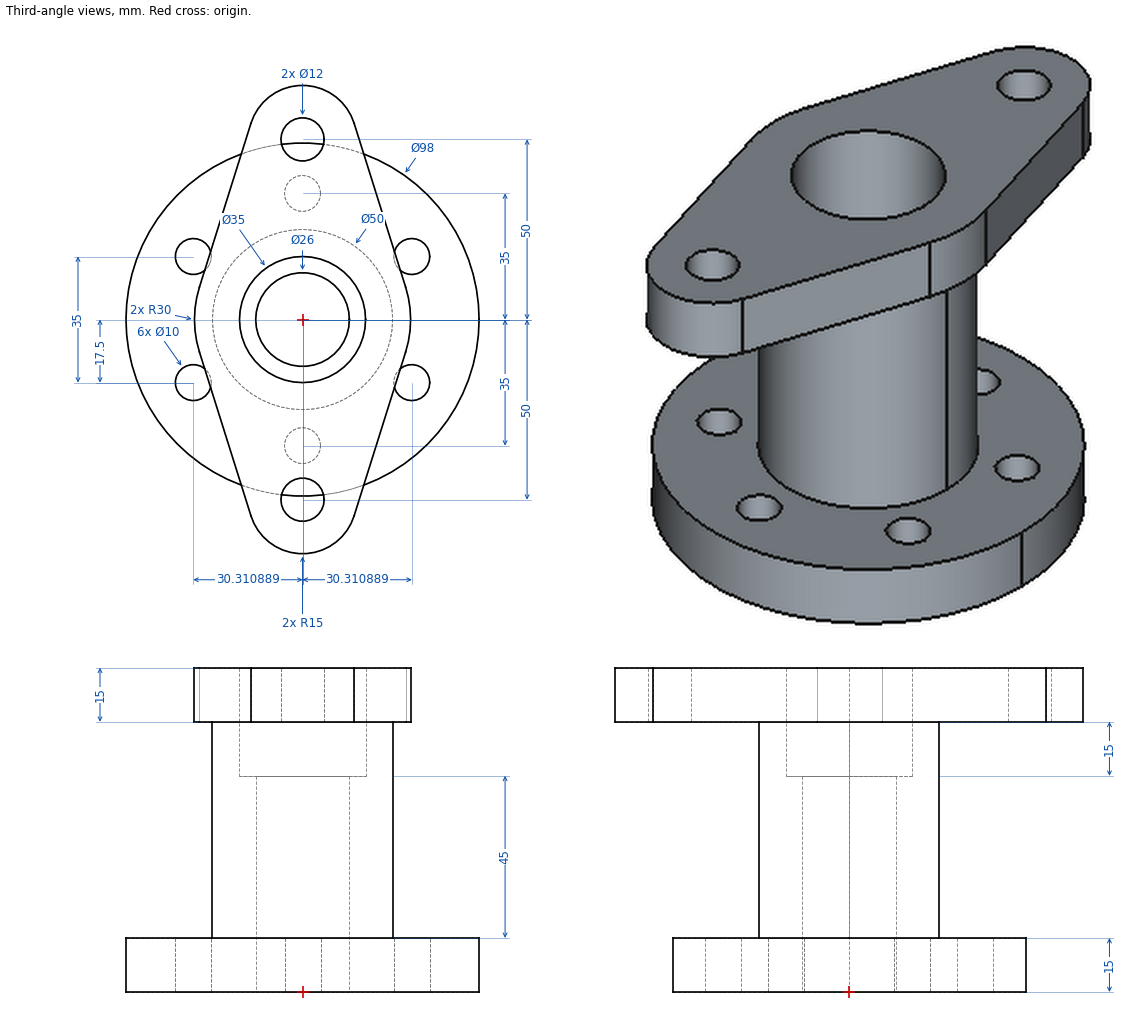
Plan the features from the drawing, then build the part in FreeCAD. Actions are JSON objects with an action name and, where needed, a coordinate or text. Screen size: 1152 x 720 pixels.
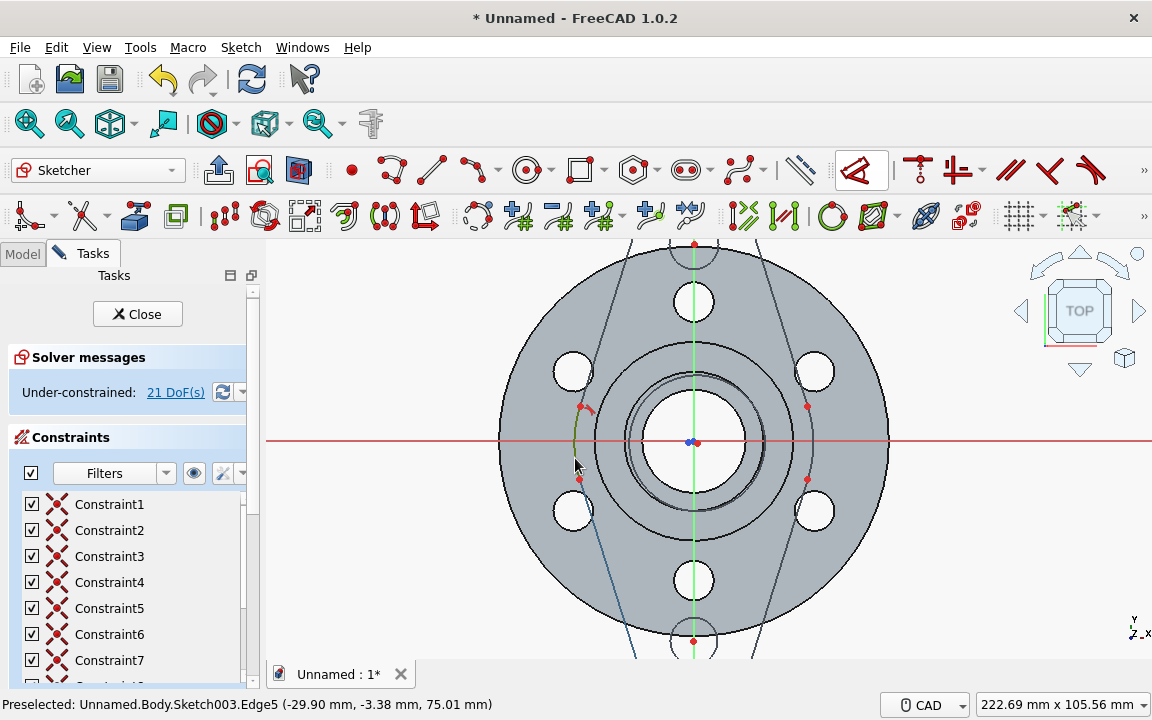
{"action": "left_click", "coordinate": [1092, 170]}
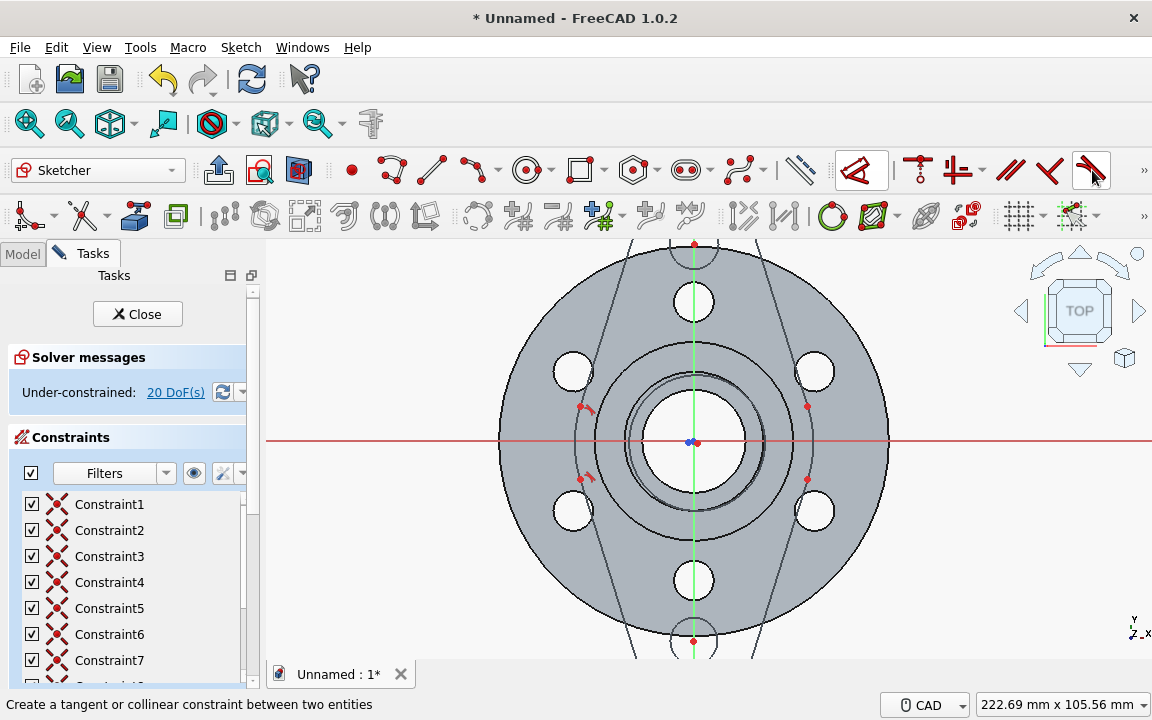
{"action": "left_click", "coordinate": [597, 534]}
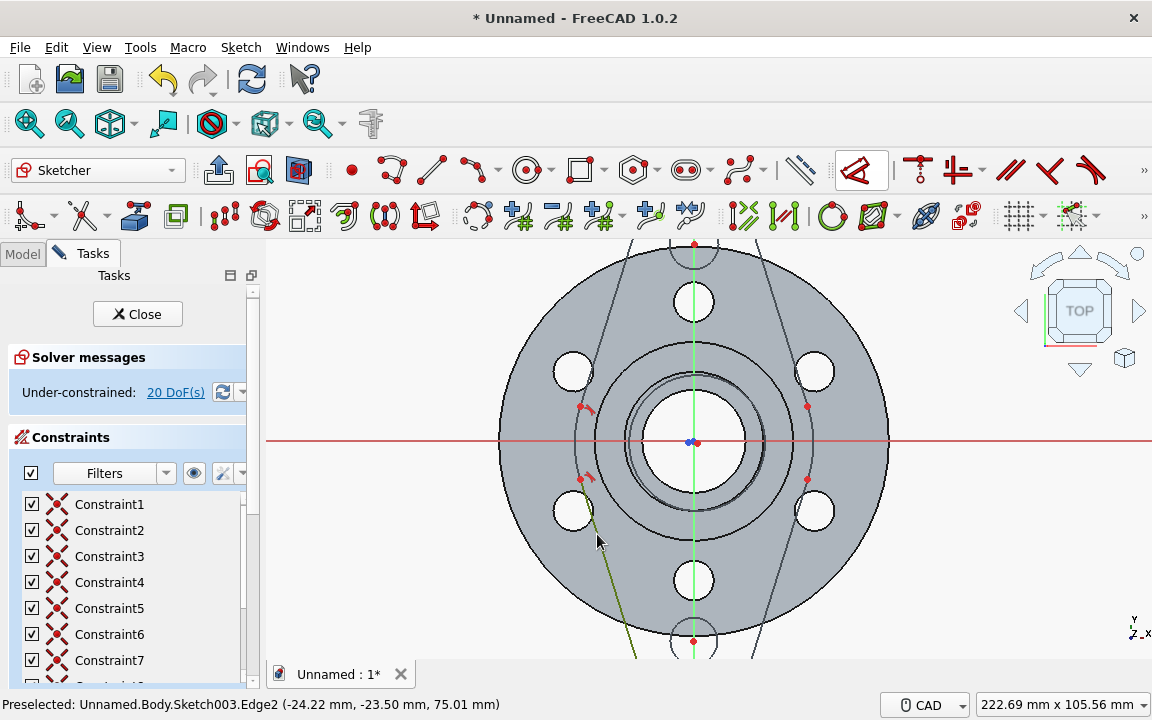
{"action": "scroll", "coordinate": [576, 458], "scroll_direction": "down", "scroll_amount": 3}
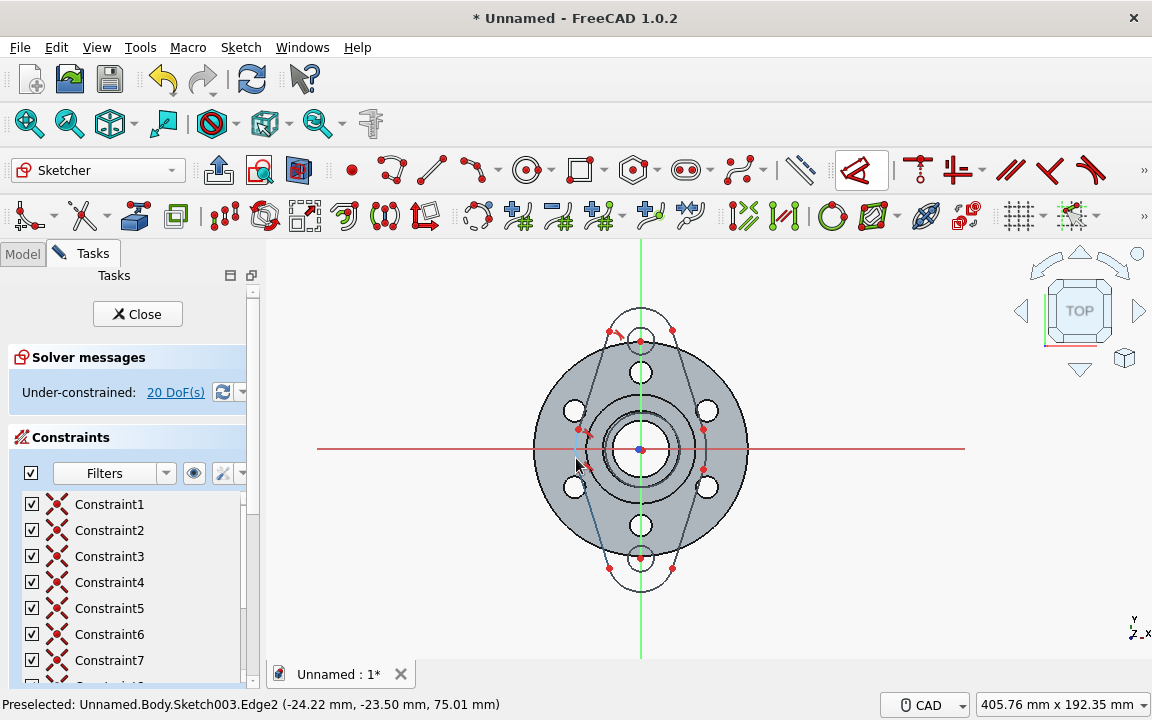
{"action": "left_click", "coordinate": [625, 588]}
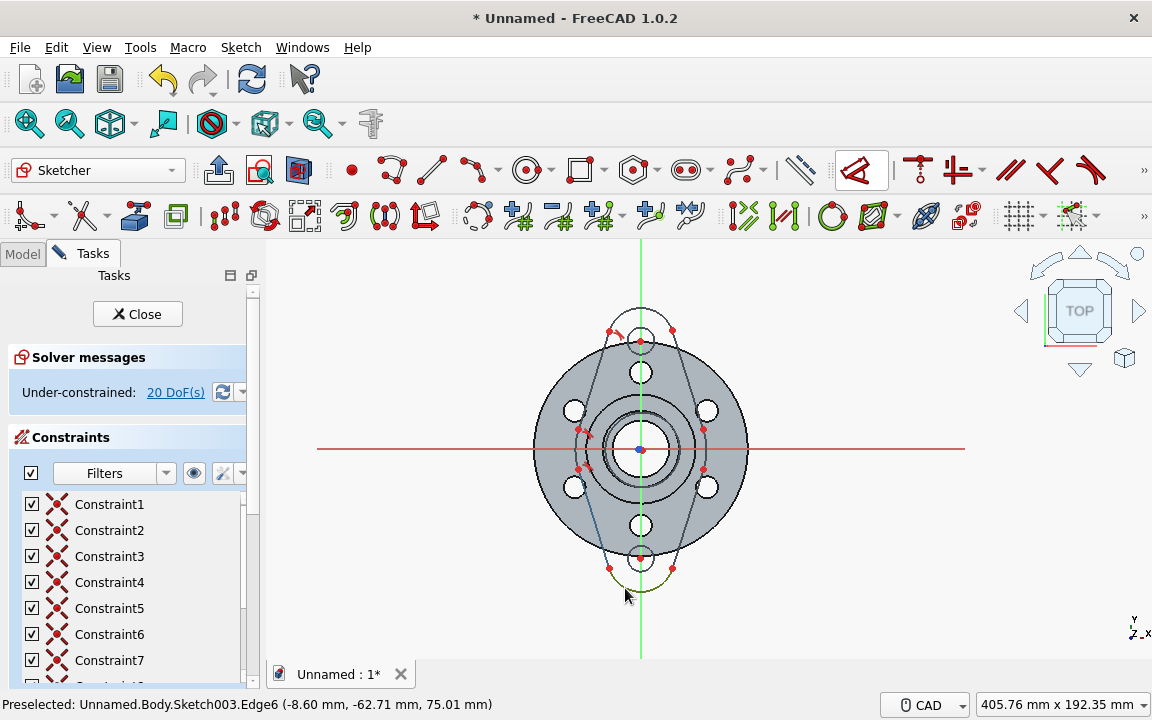
{"action": "key", "text": "t"}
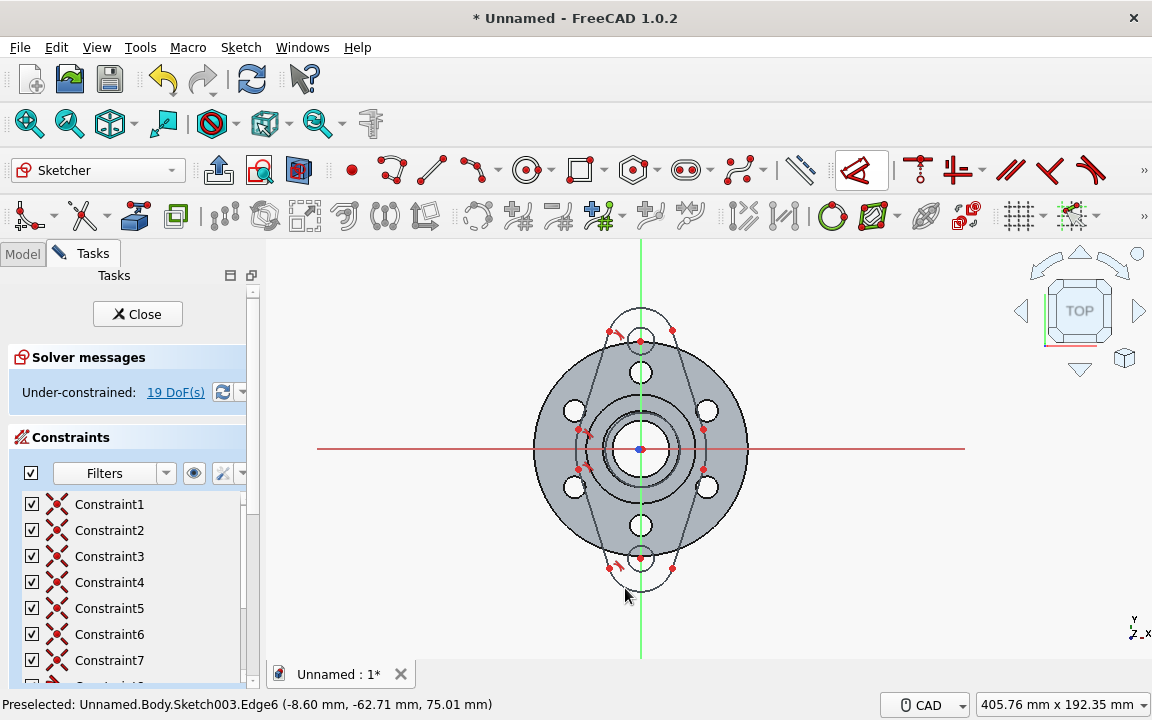
{"action": "left_click", "coordinate": [682, 539]}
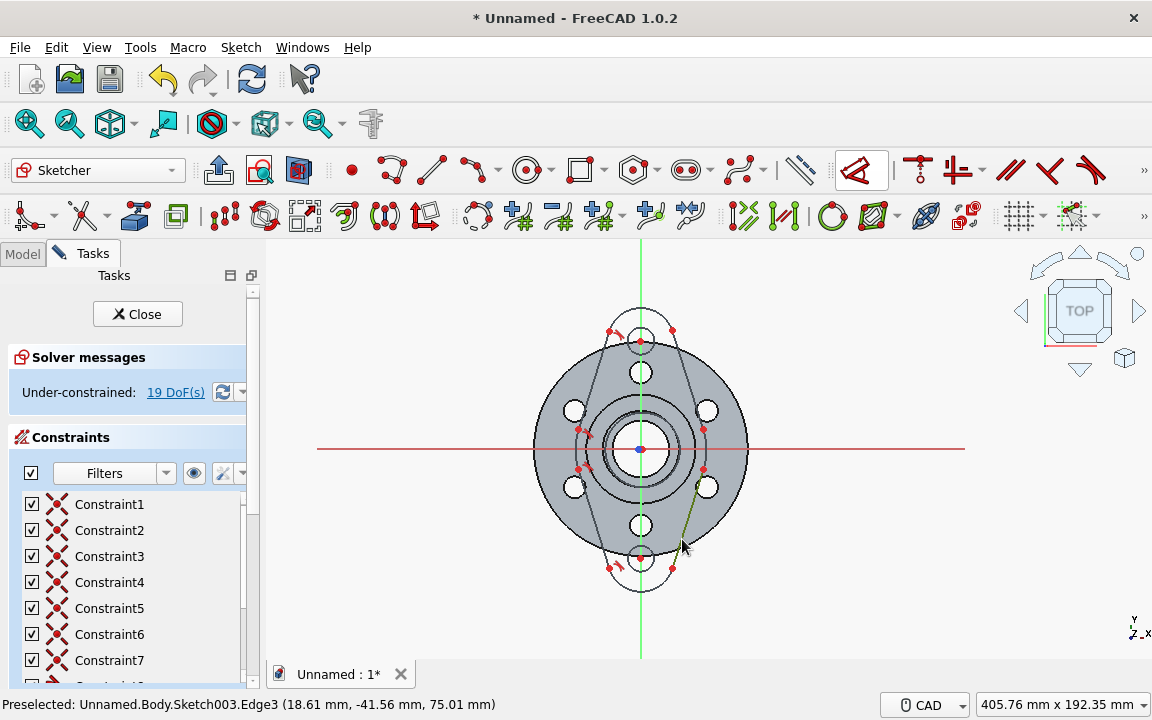
{"action": "left_click", "coordinate": [625, 588]}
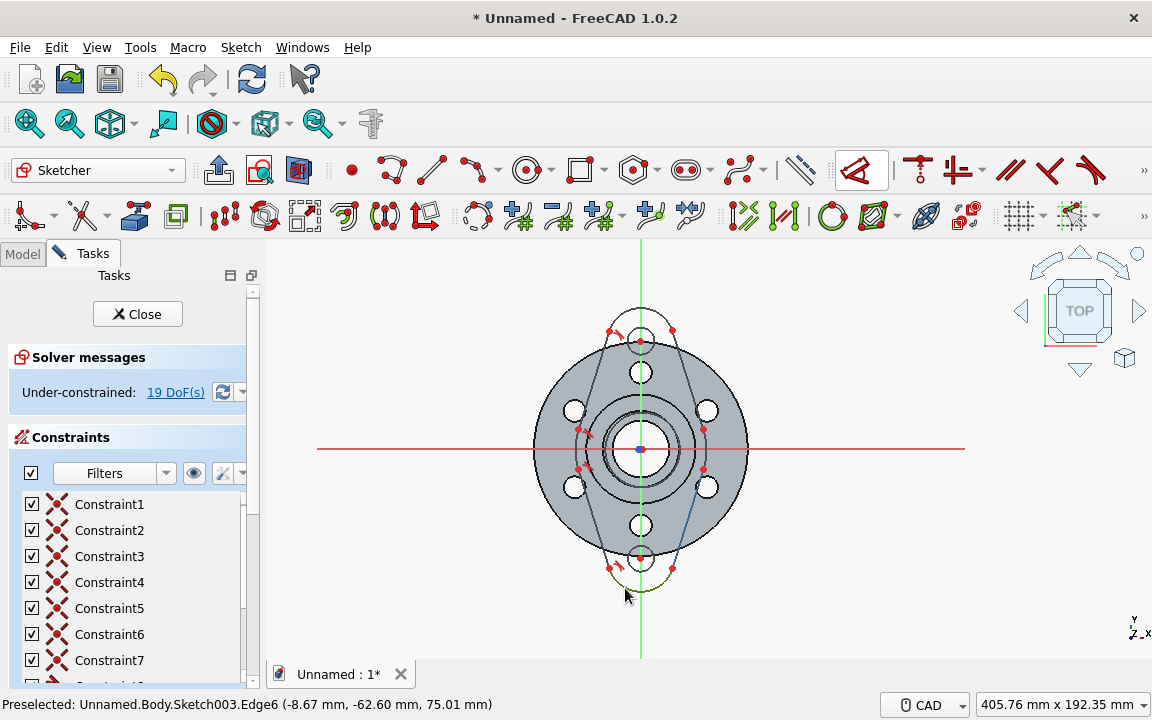
{"action": "key", "text": "t"}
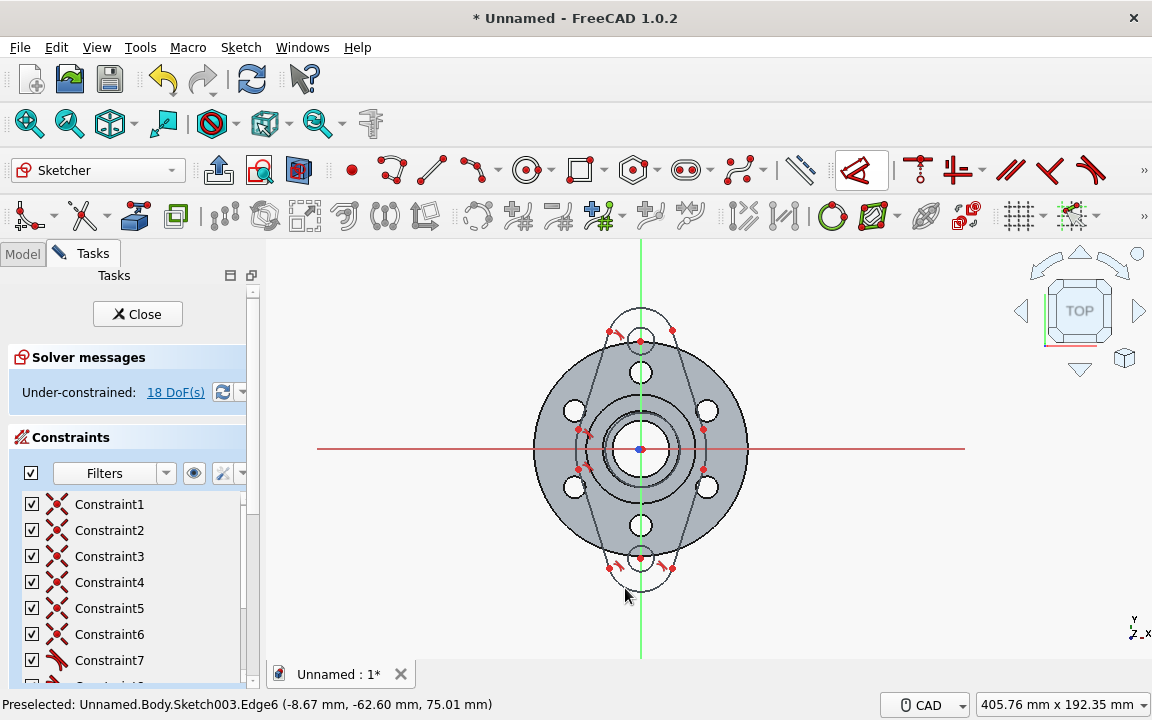
{"action": "left_click", "coordinate": [682, 539]}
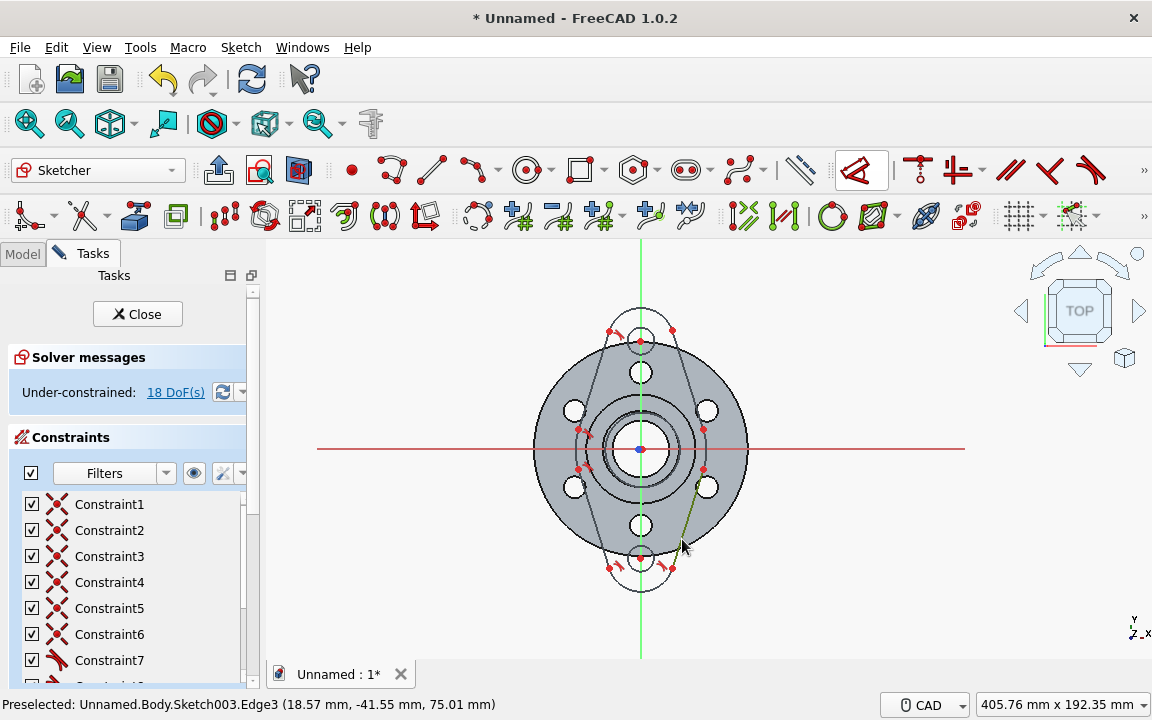
{"action": "scroll", "coordinate": [706, 458], "scroll_direction": "up", "scroll_amount": 3}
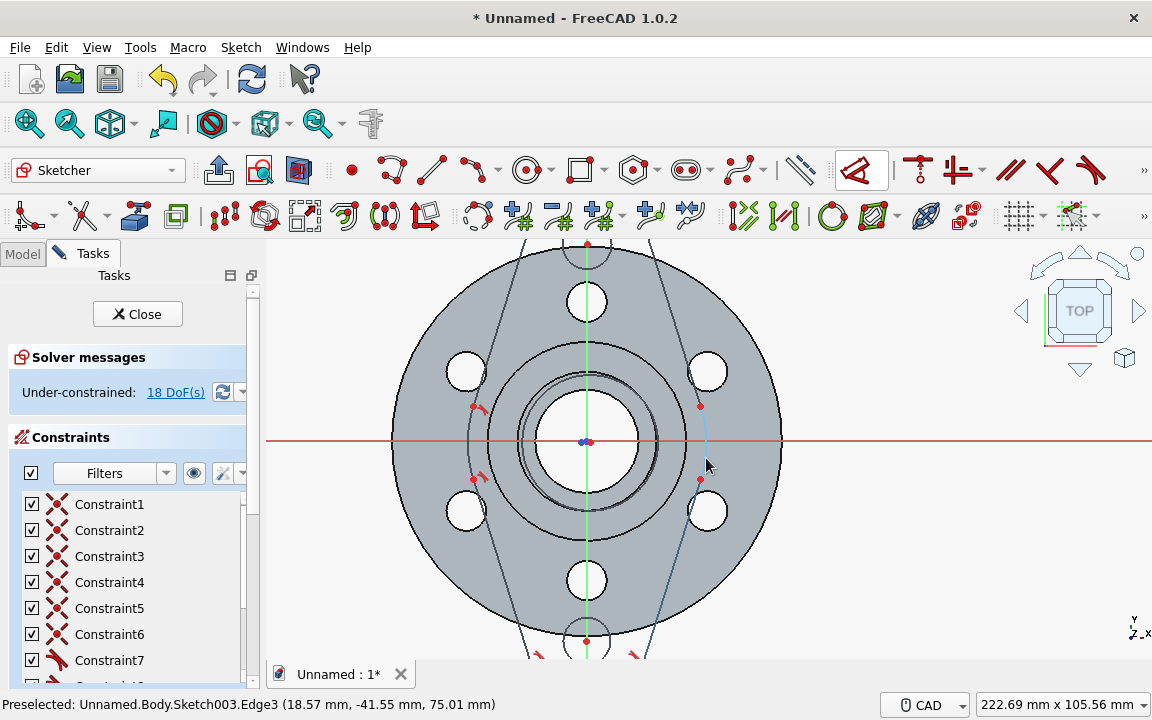
{"action": "left_click", "coordinate": [705, 458]}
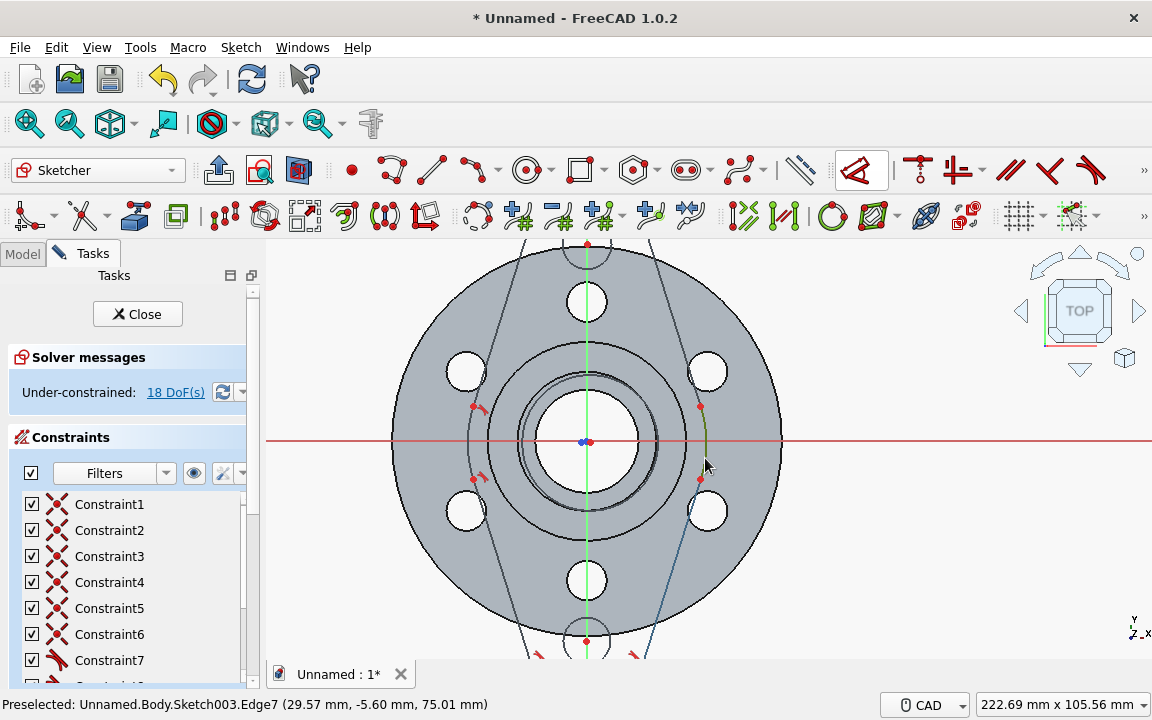
{"action": "key", "text": "t"}